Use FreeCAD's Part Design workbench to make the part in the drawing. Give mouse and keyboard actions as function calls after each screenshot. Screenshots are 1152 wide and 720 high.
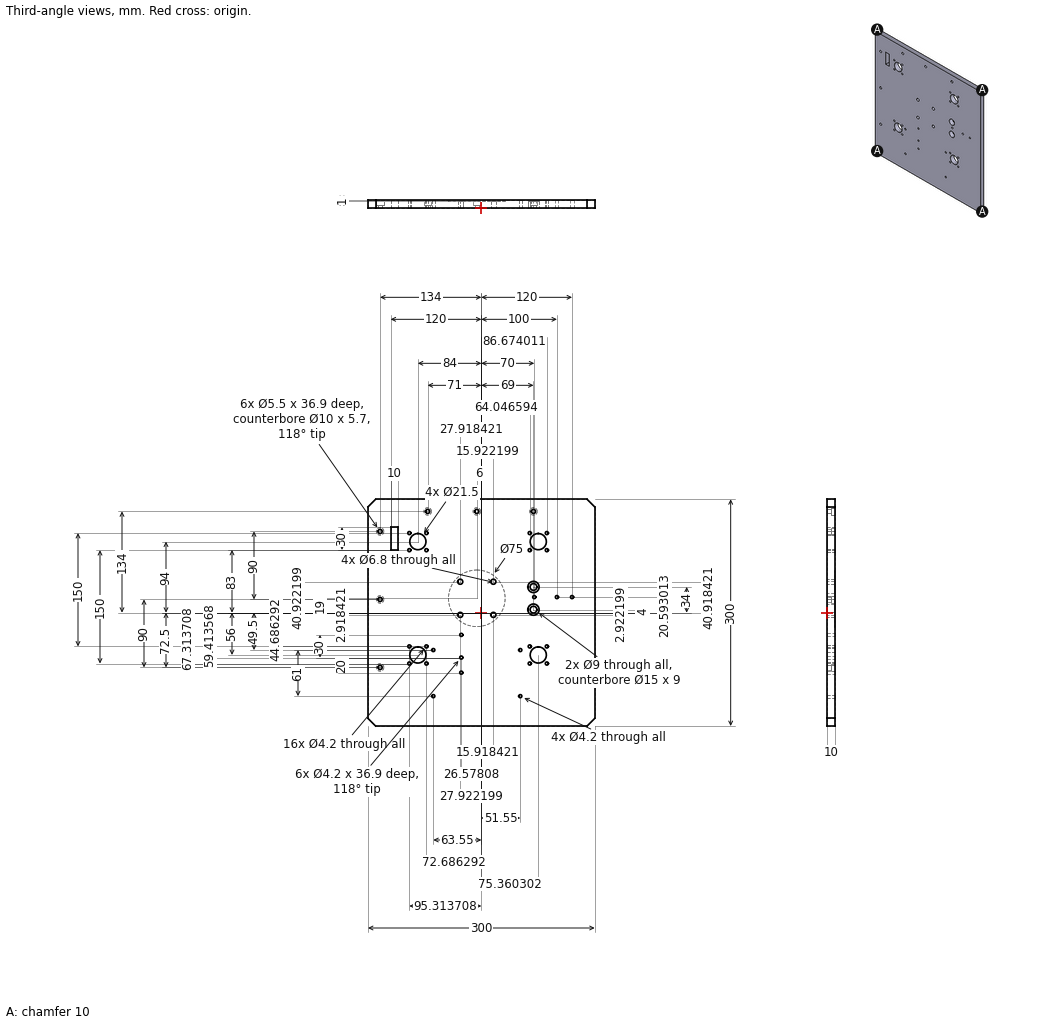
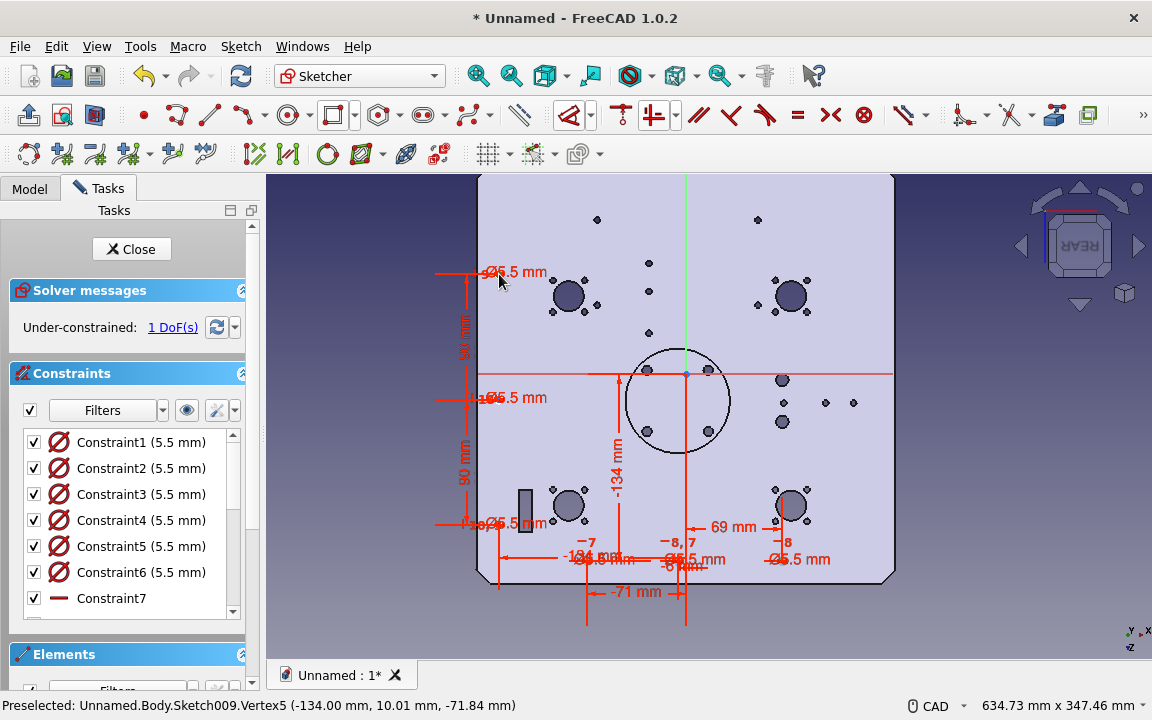
key(i)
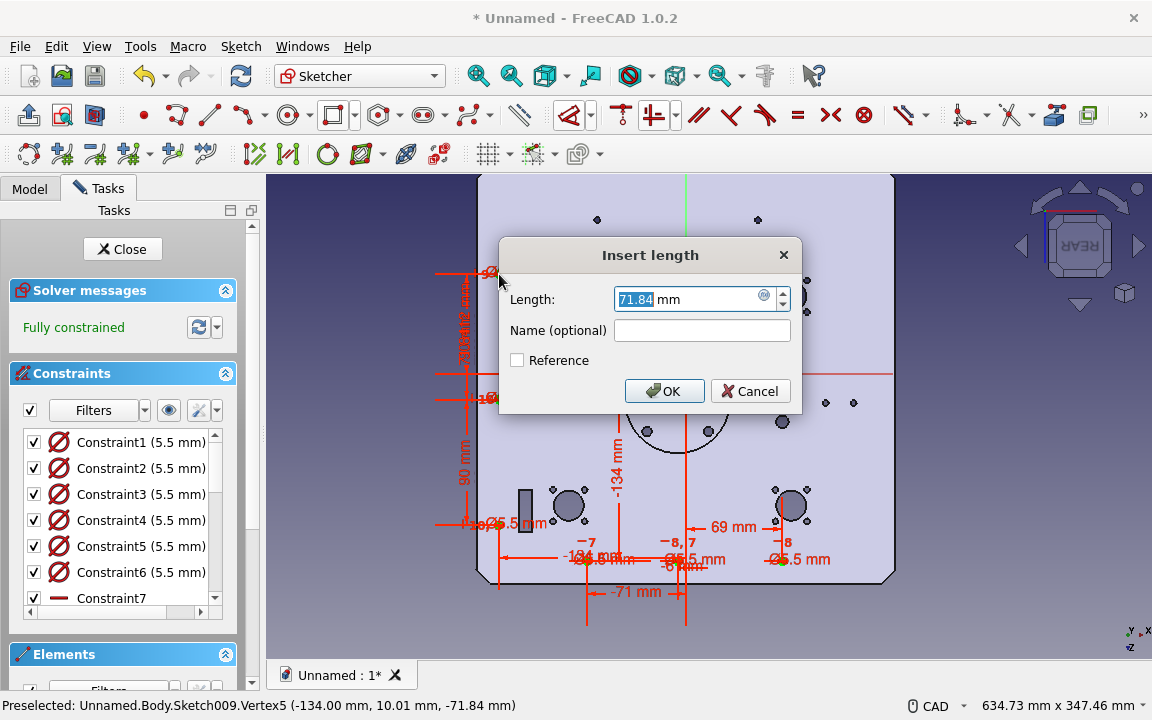
text(72.5)
key(Return)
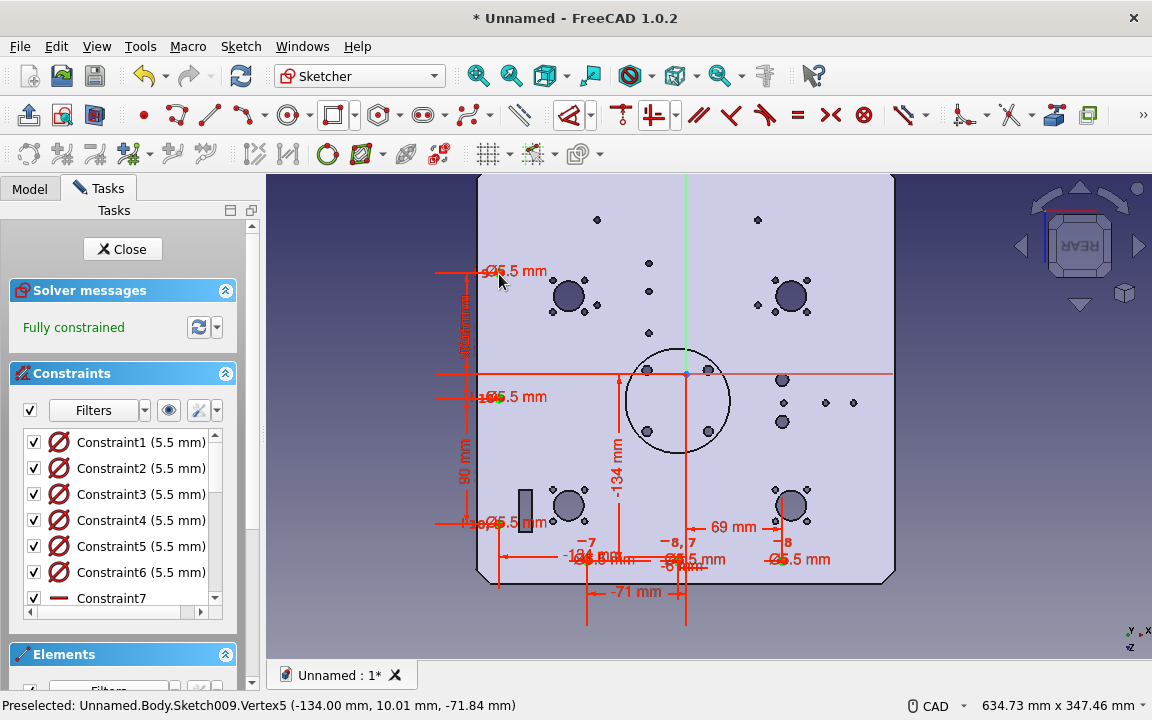
click(123, 249)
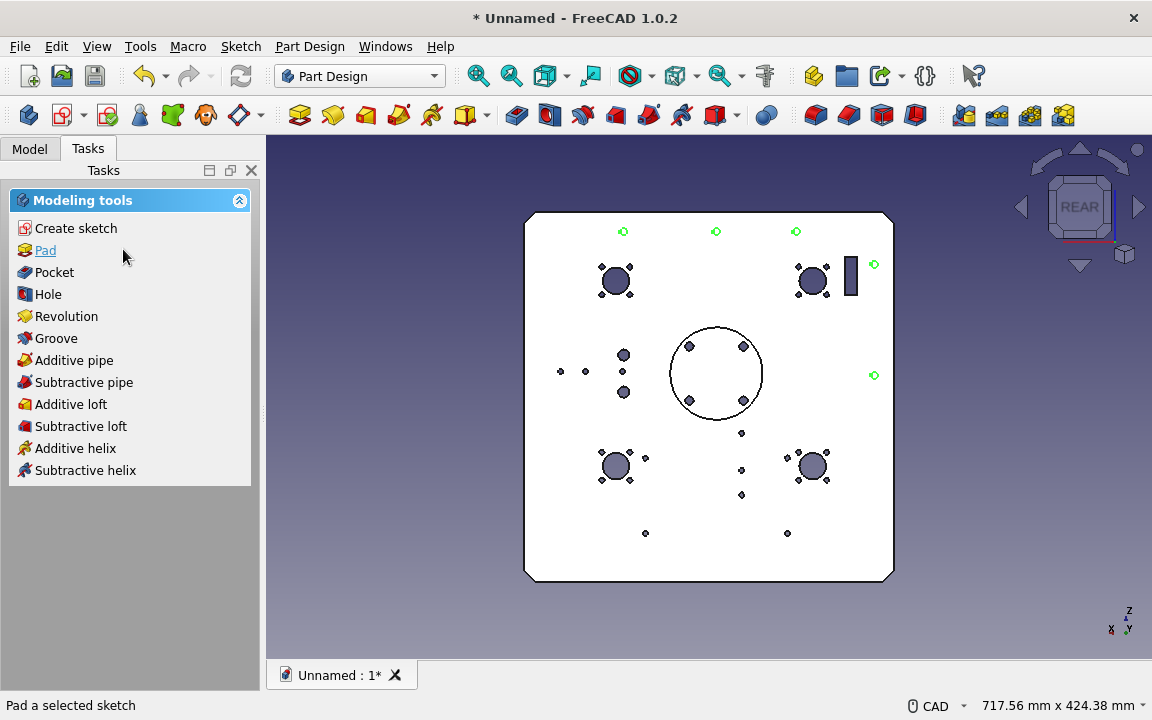
click(550, 116)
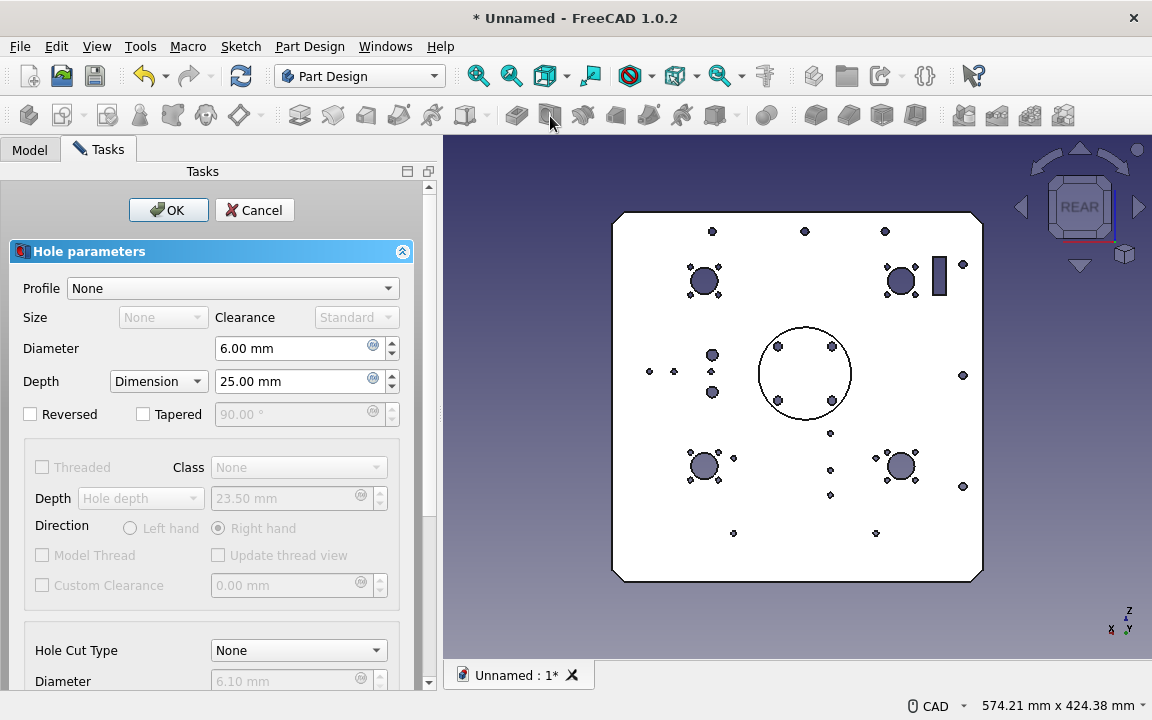
triple_click(300, 348)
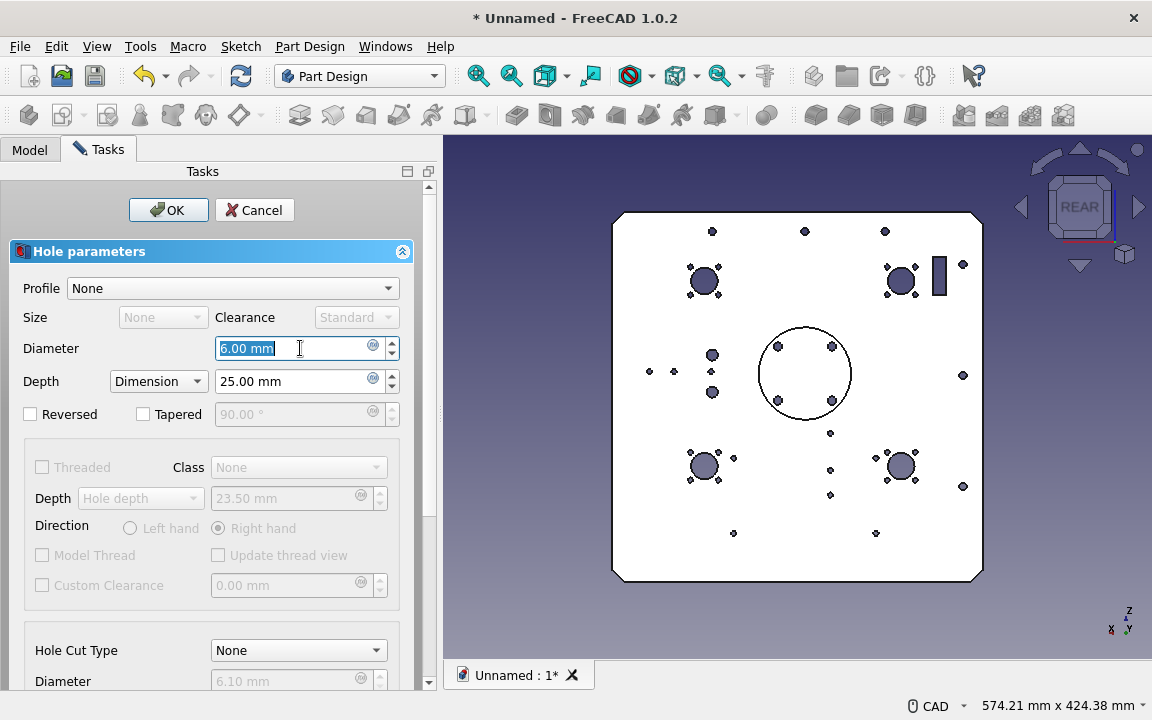
text(5.5)
key(Tab)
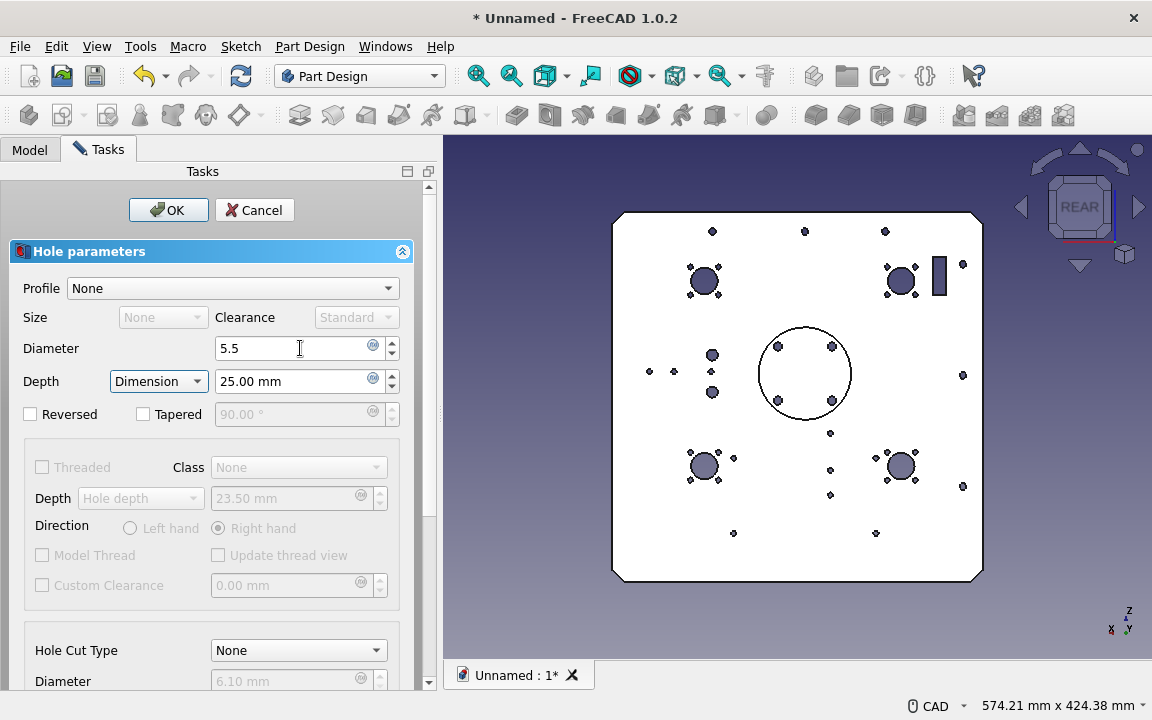
triple_click(300, 382)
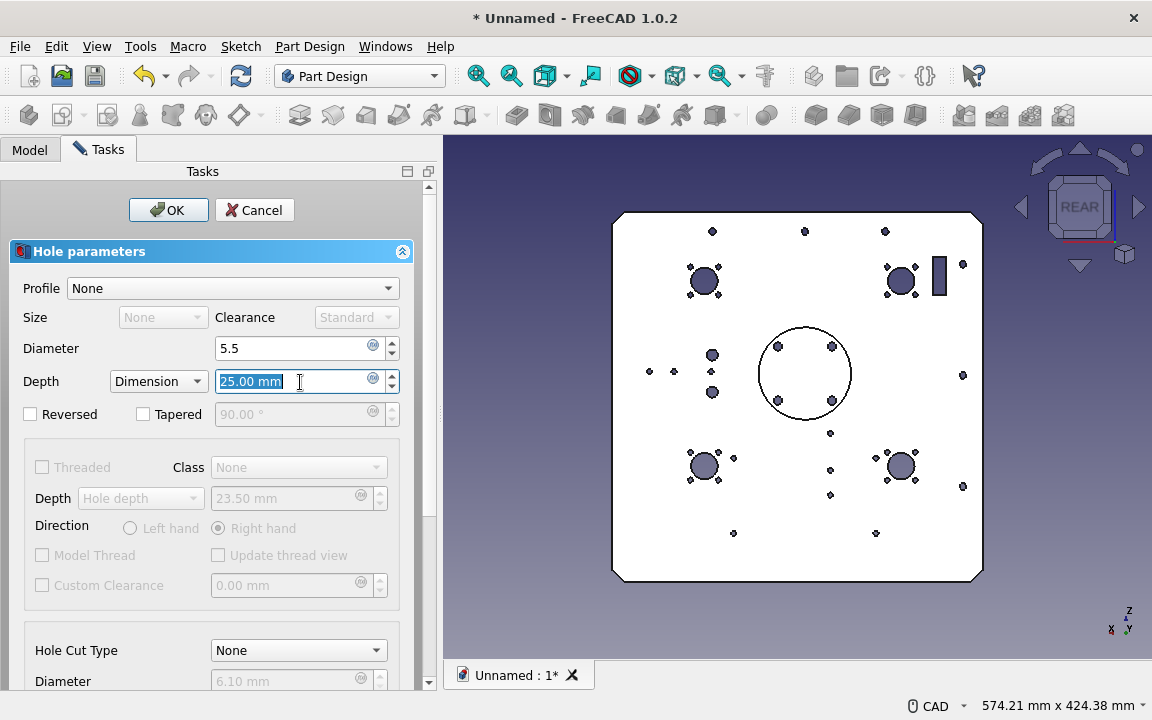
text(36.9)
key(Tab)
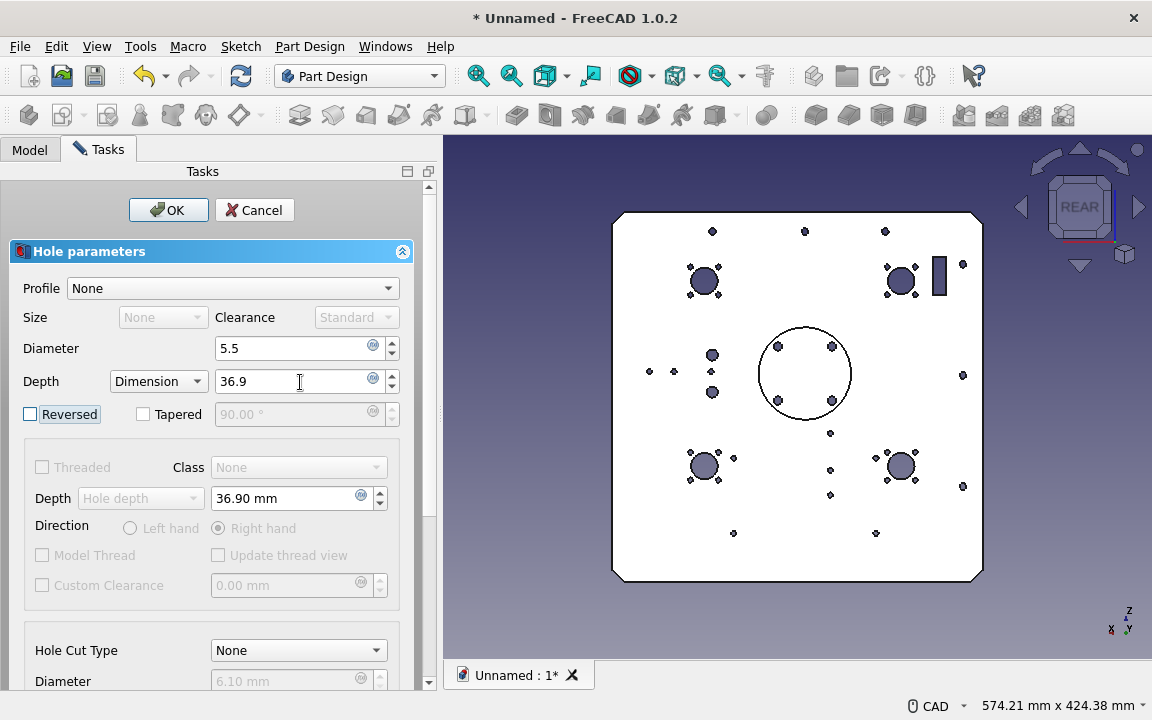
click(300, 650)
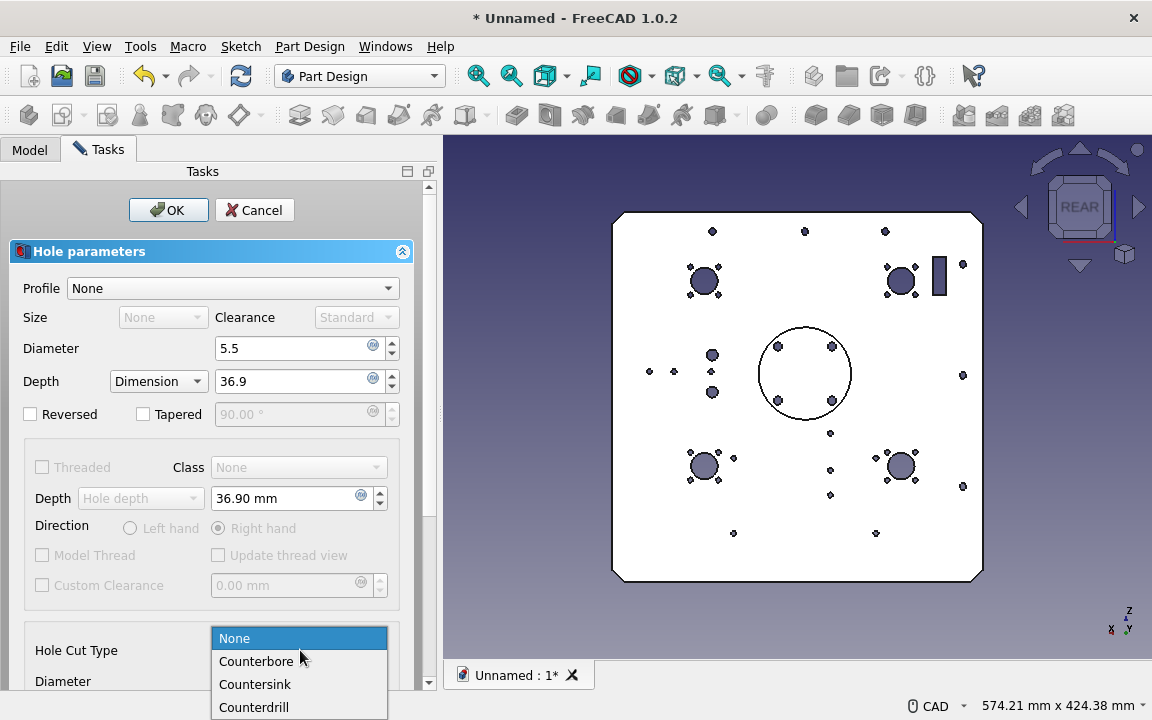
click(298, 662)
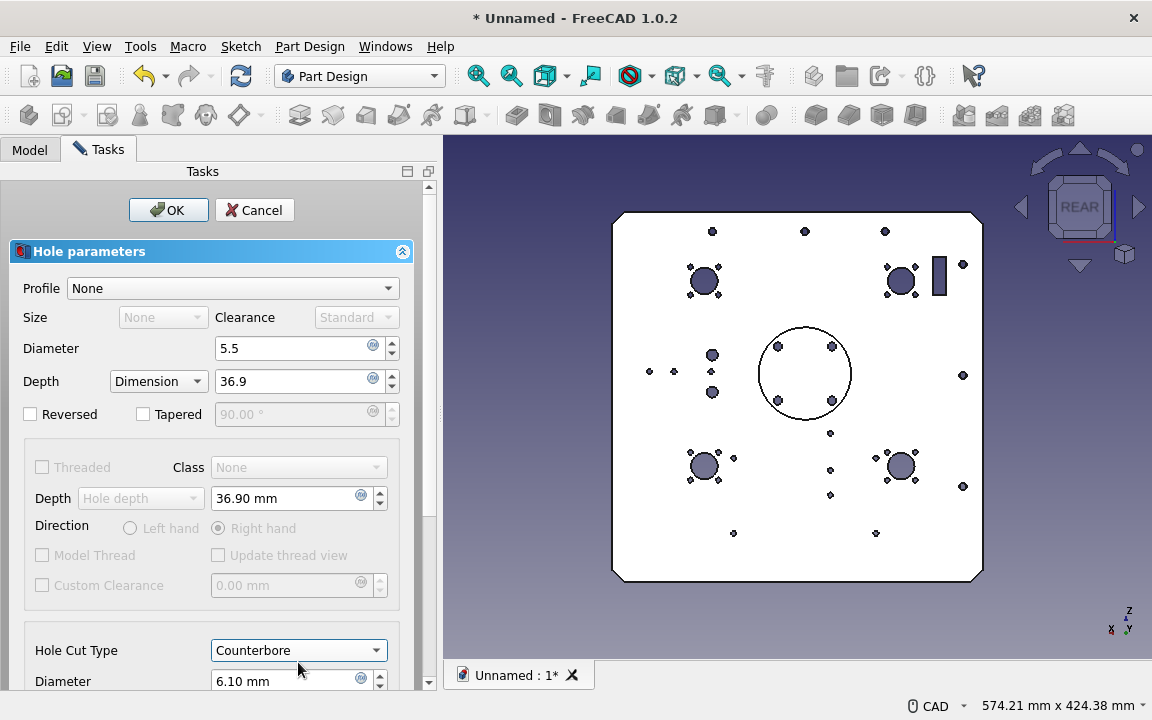
scroll(429, 436, down, 2)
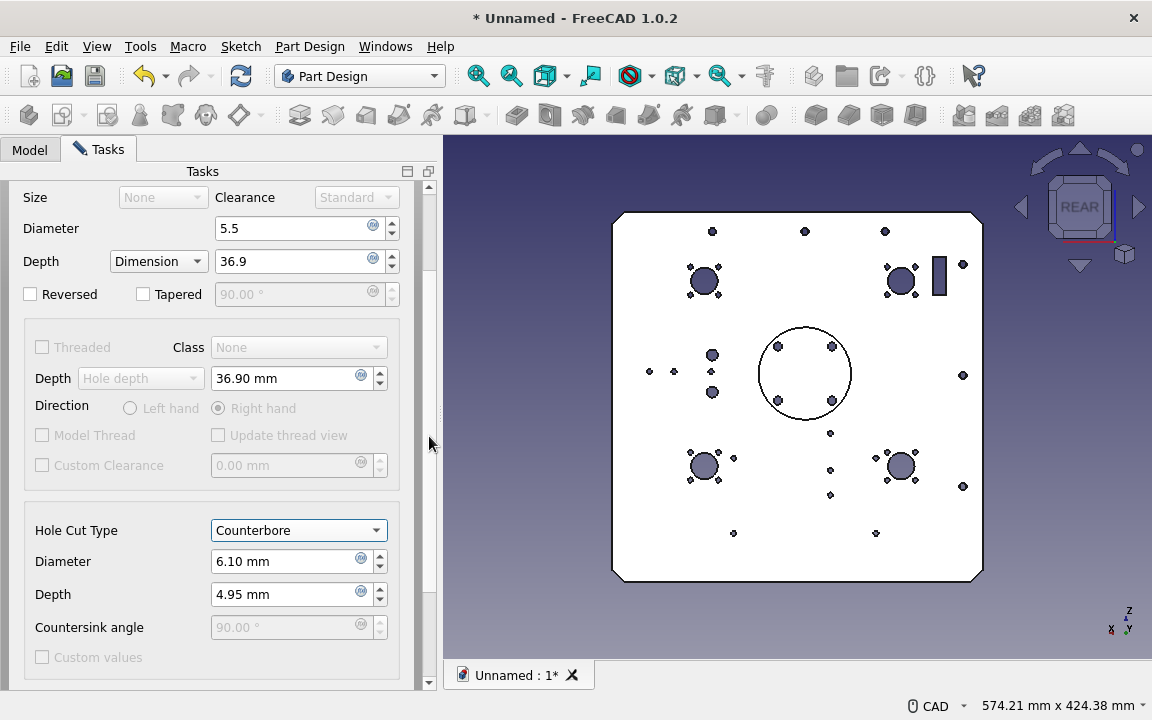
triple_click(292, 562)